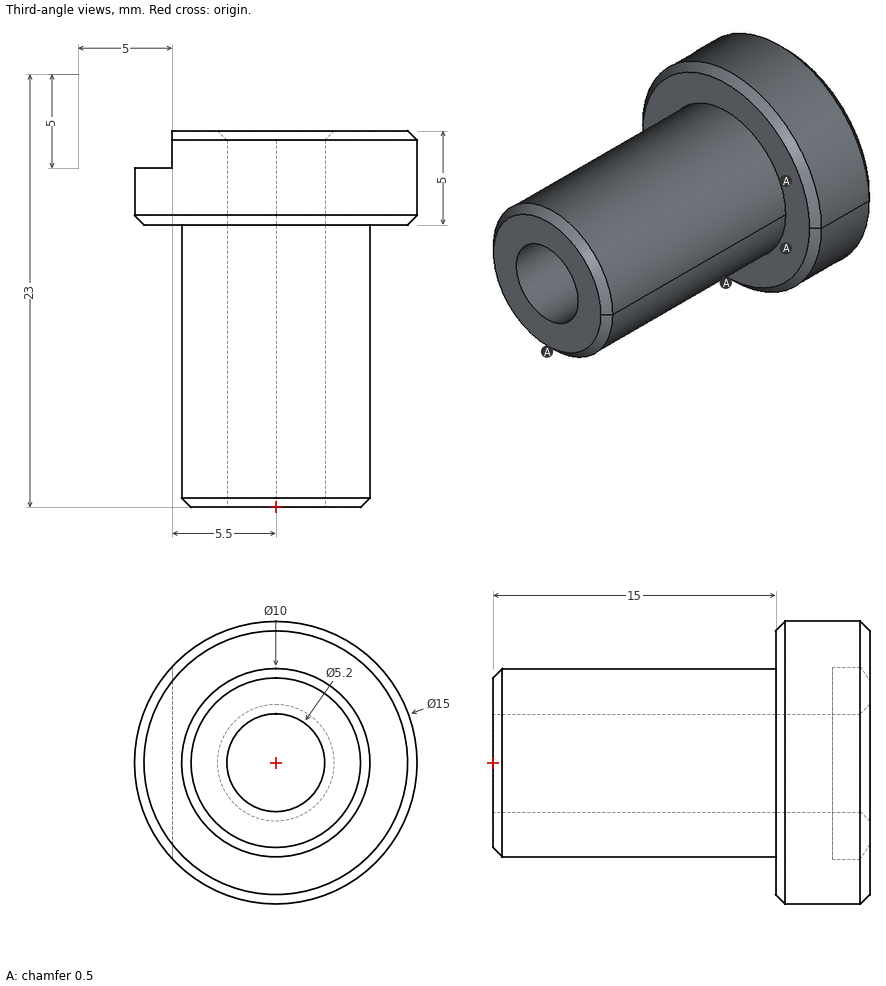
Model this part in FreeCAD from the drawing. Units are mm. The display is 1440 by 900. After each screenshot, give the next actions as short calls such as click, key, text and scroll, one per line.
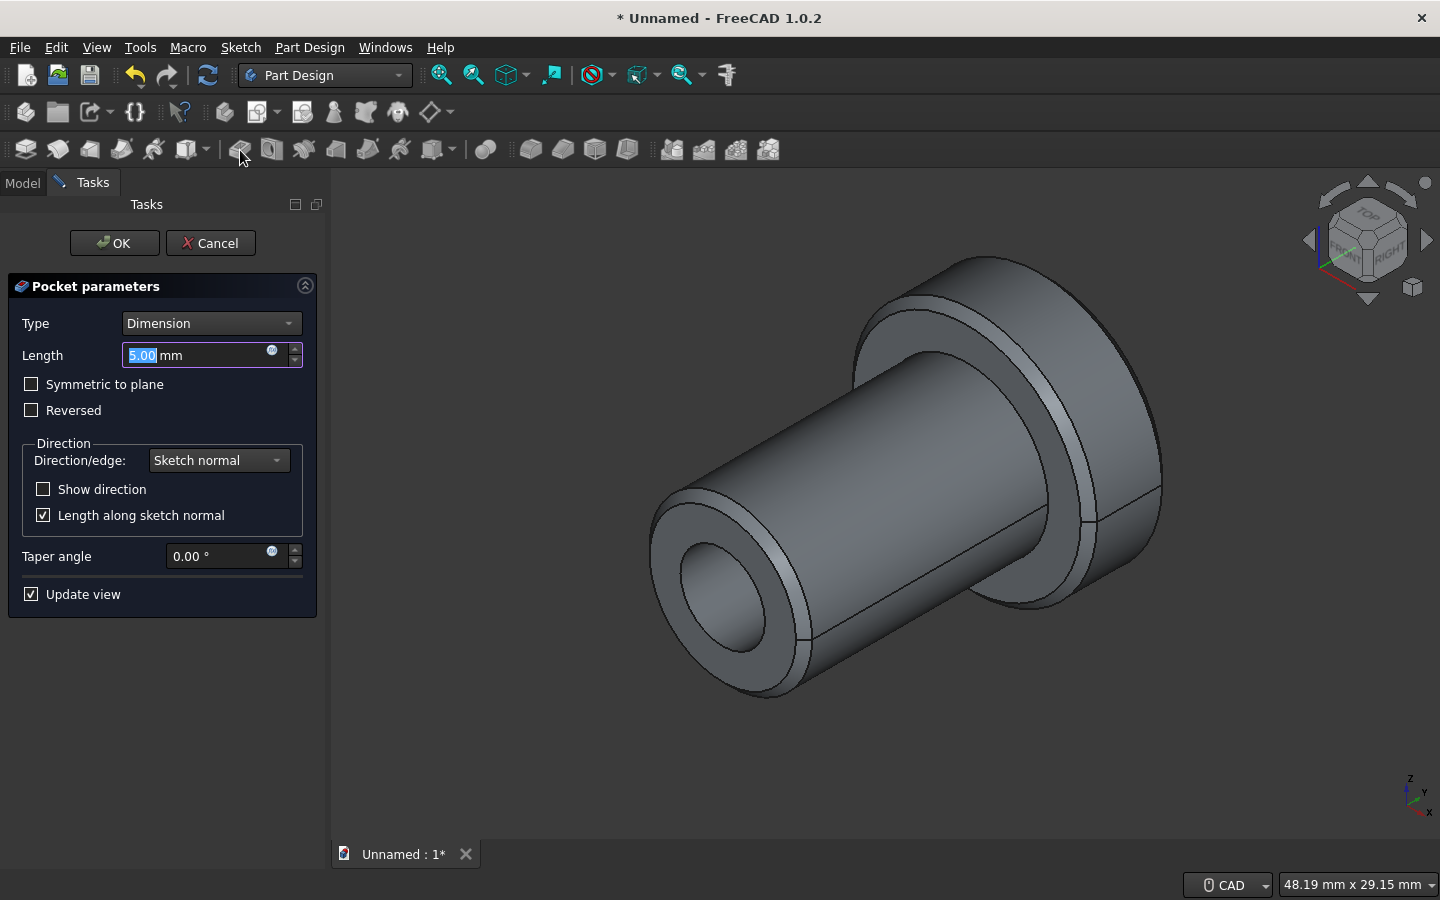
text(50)
key(Tab)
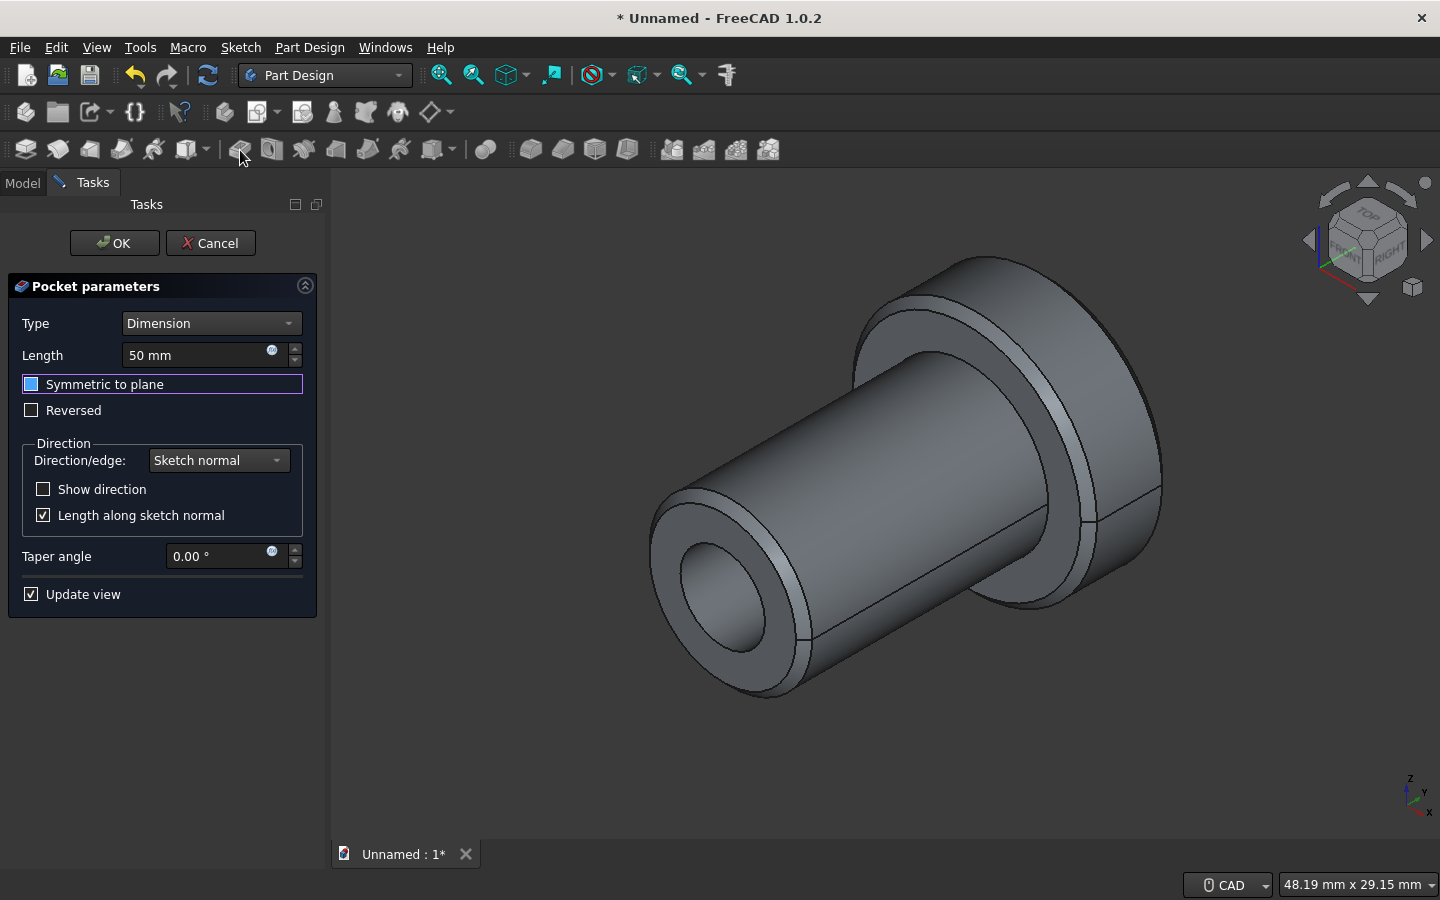
click(30, 384)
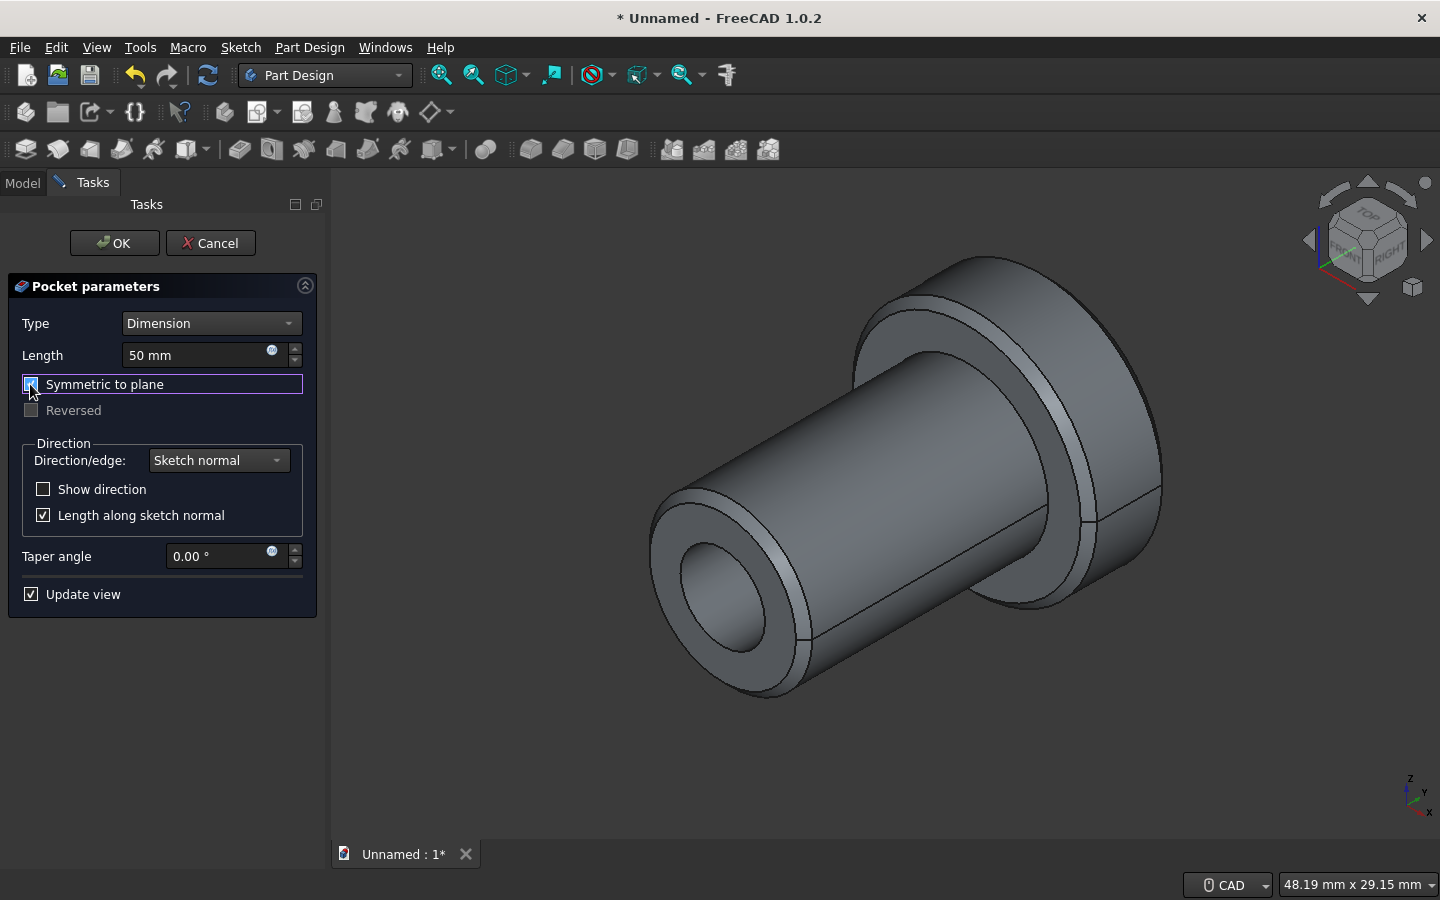
click(115, 243)